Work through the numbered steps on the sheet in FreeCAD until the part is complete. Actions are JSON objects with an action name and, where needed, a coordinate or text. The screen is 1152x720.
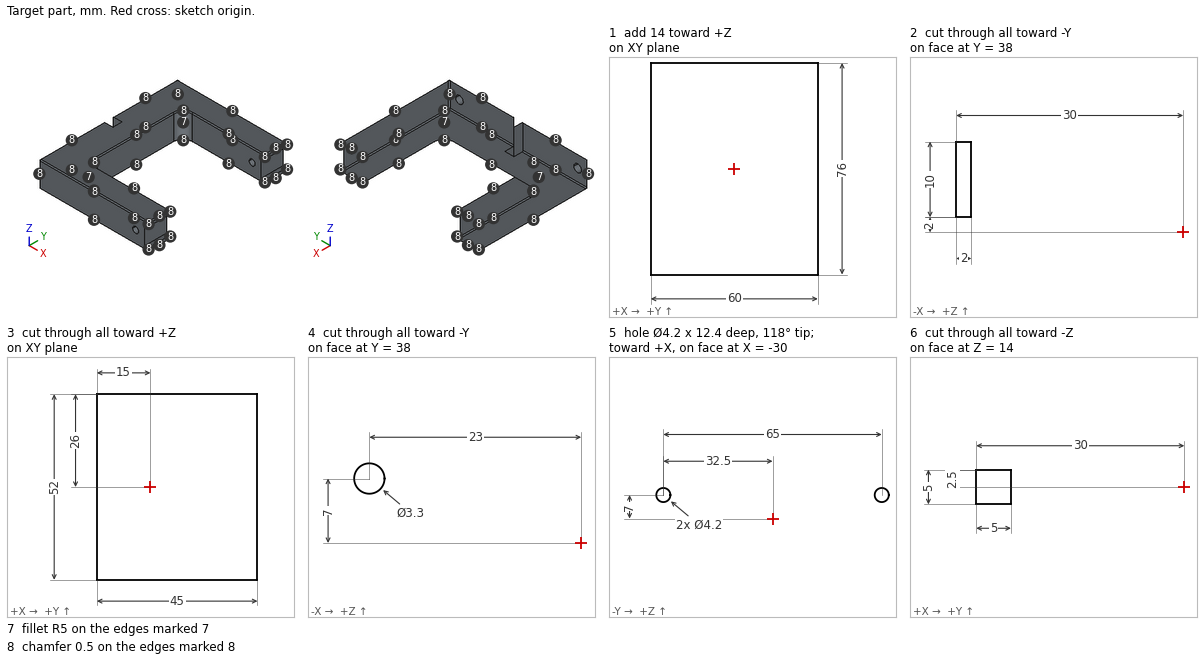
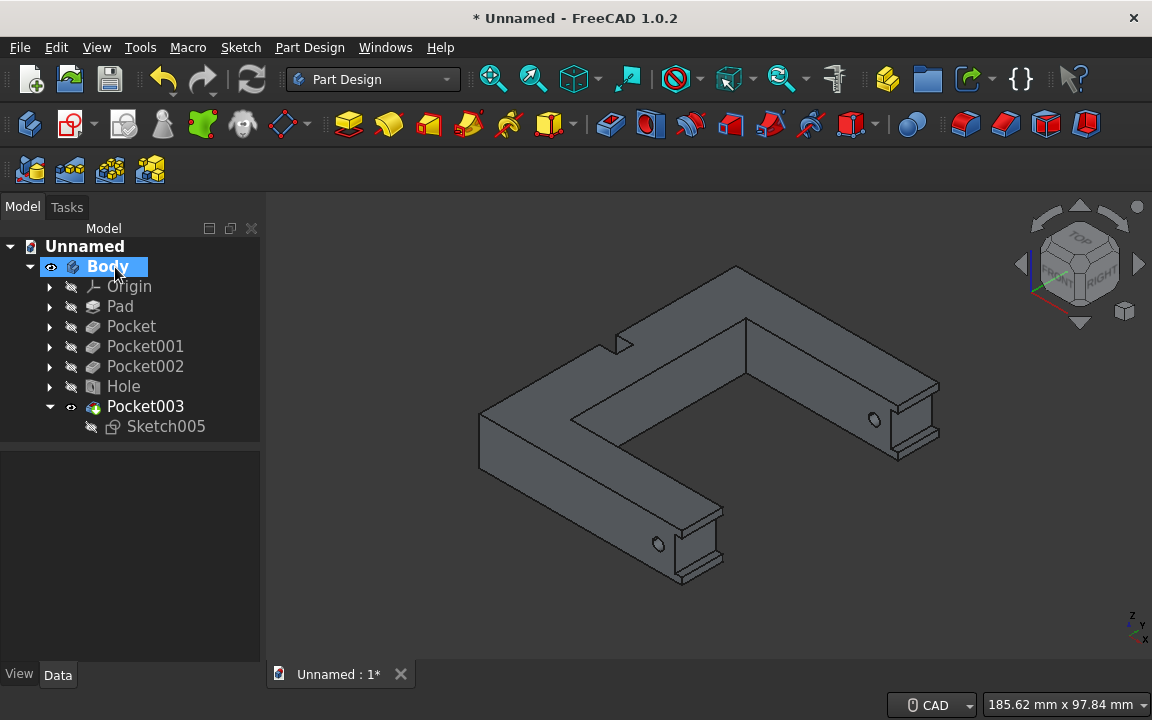
{"action": "key", "text": "1"}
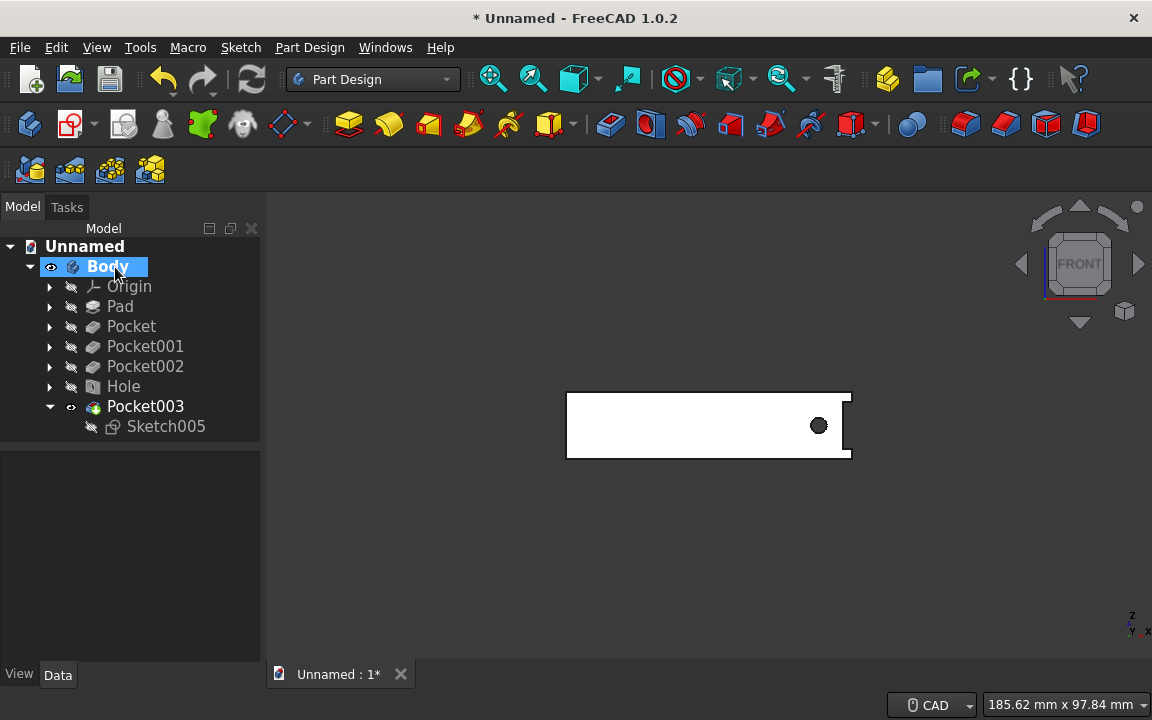
{"action": "key", "text": "v f"}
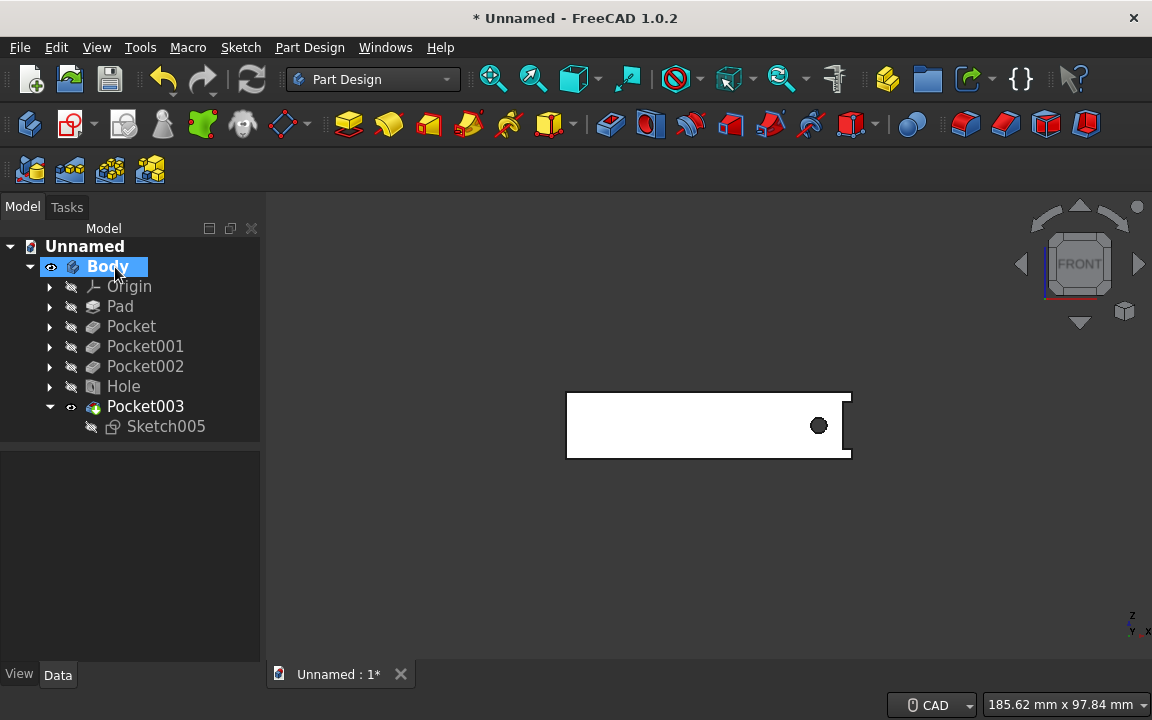
{"action": "key", "text": "3"}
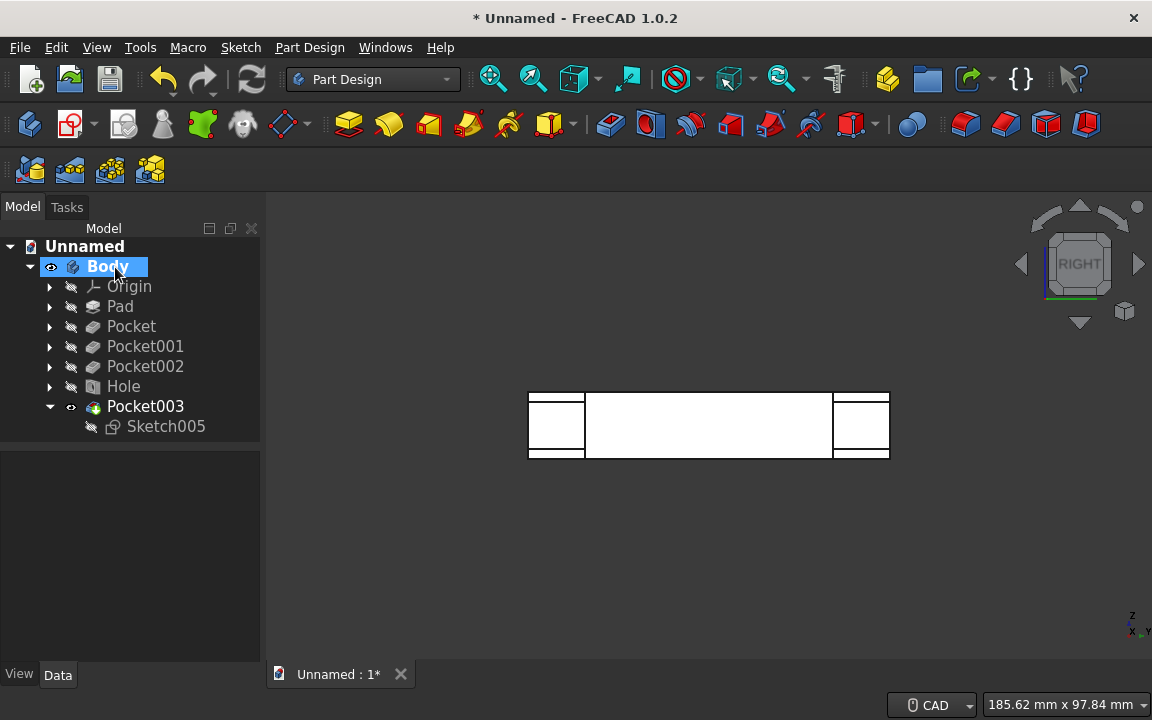
{"action": "key", "text": "v f"}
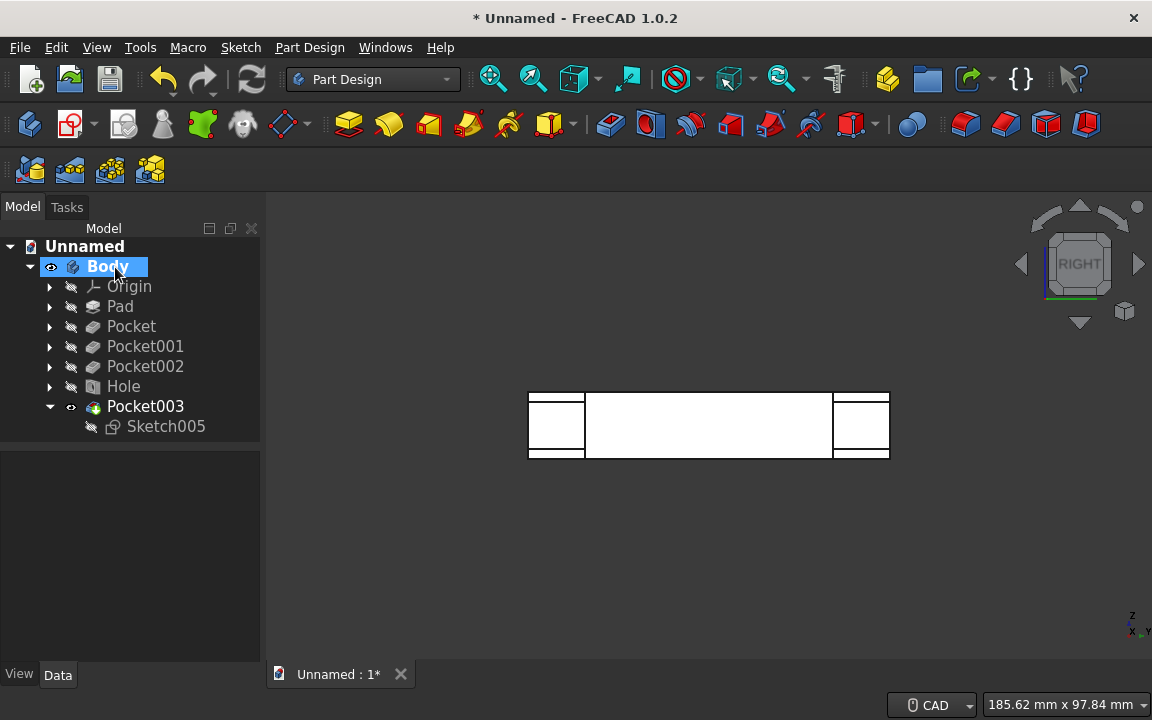
{"action": "key", "text": "5"}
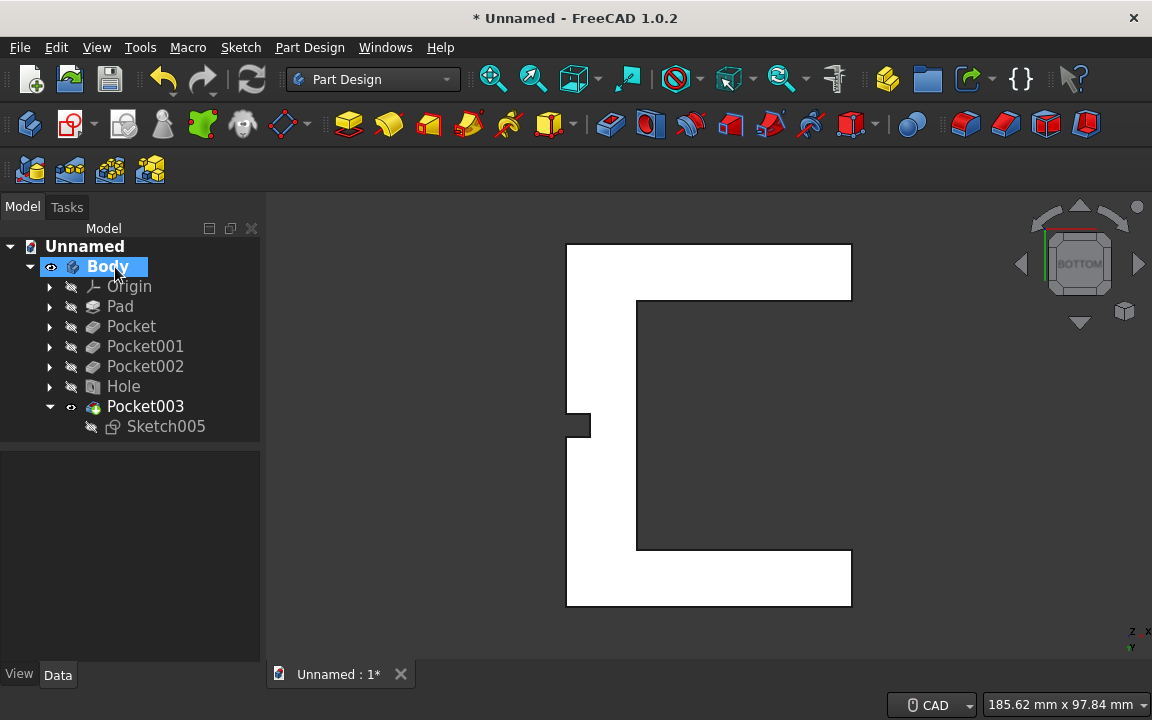
{"action": "key", "text": "4"}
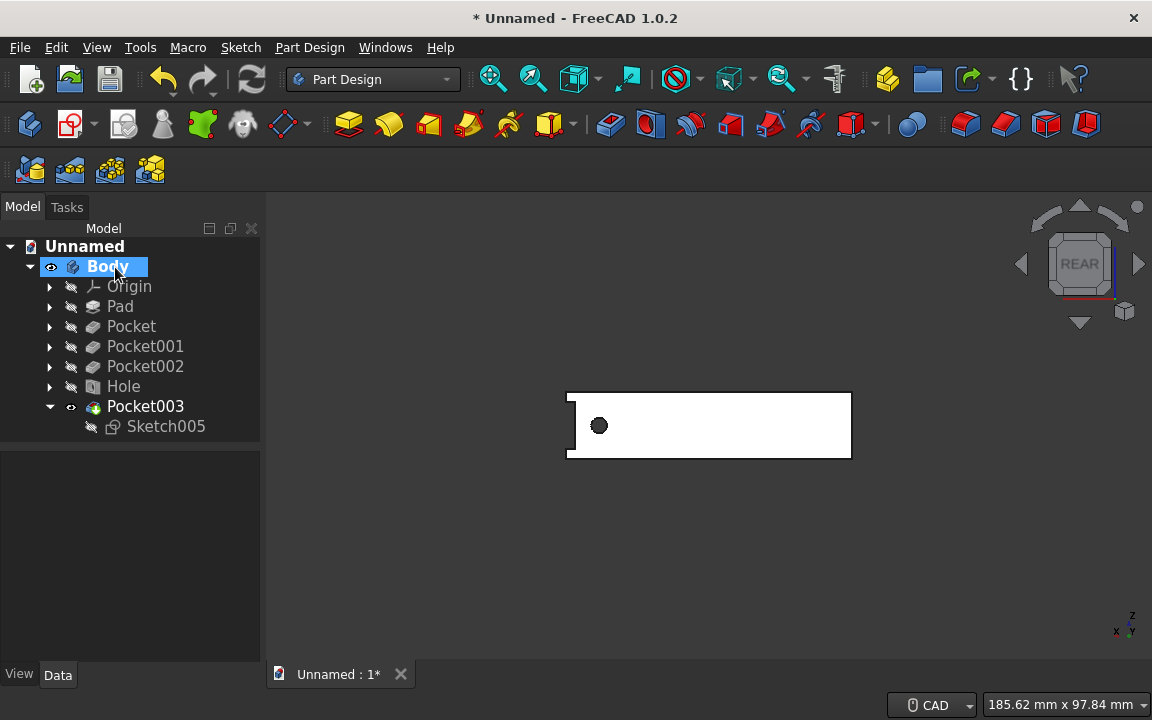
{"action": "key", "text": "v f"}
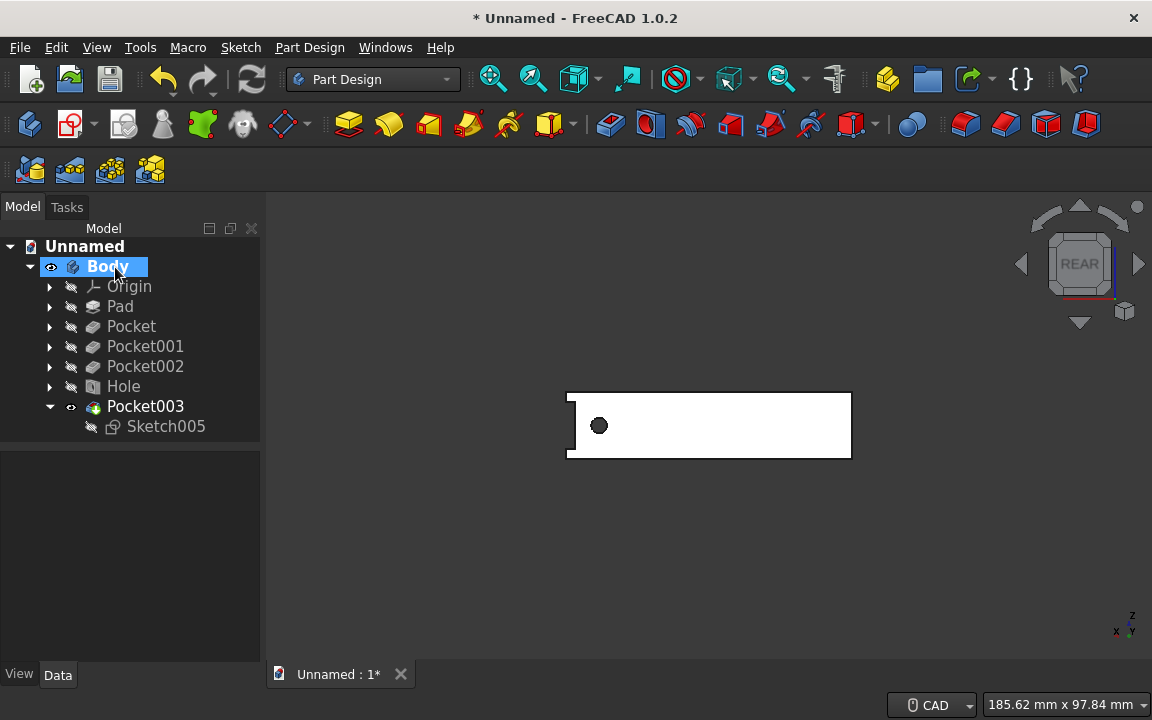
{"action": "key", "text": "6"}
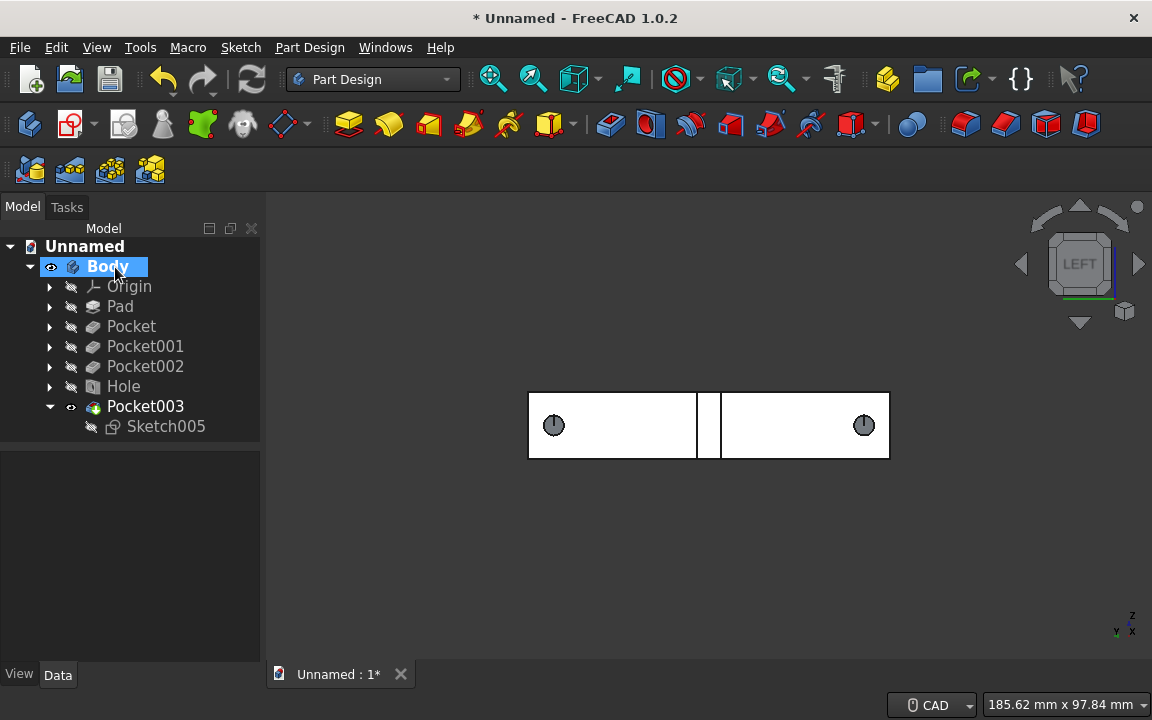
{"action": "key", "text": "v f"}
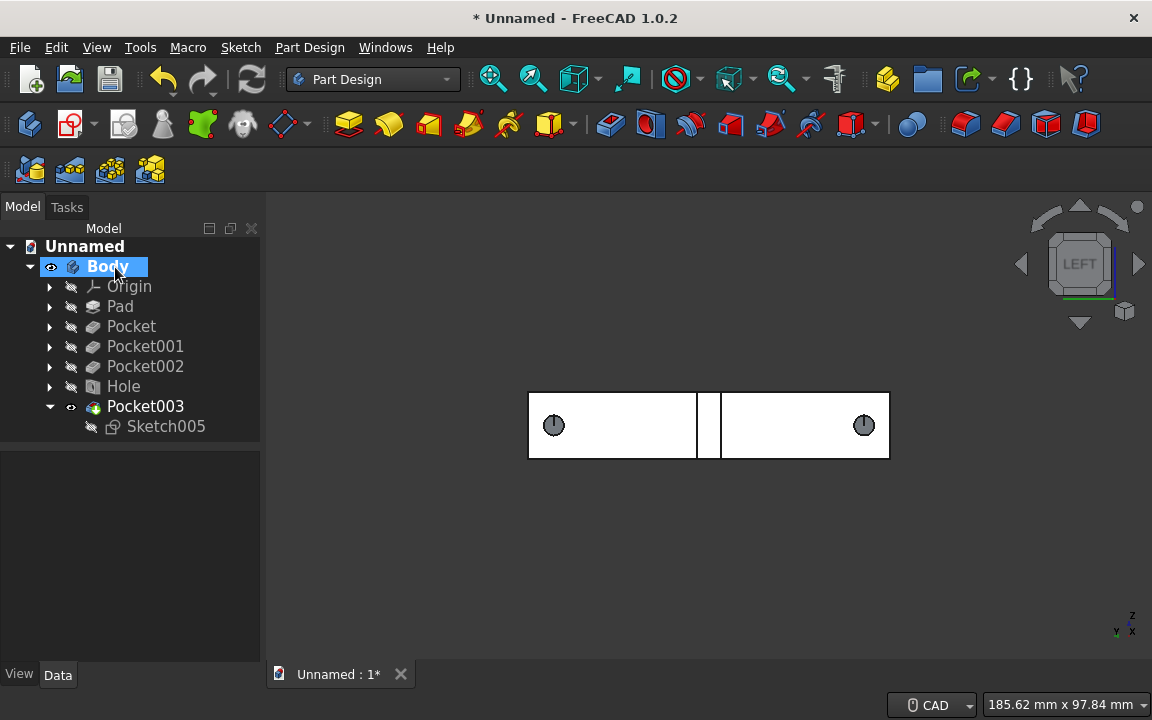
{"action": "key", "text": "v 3"}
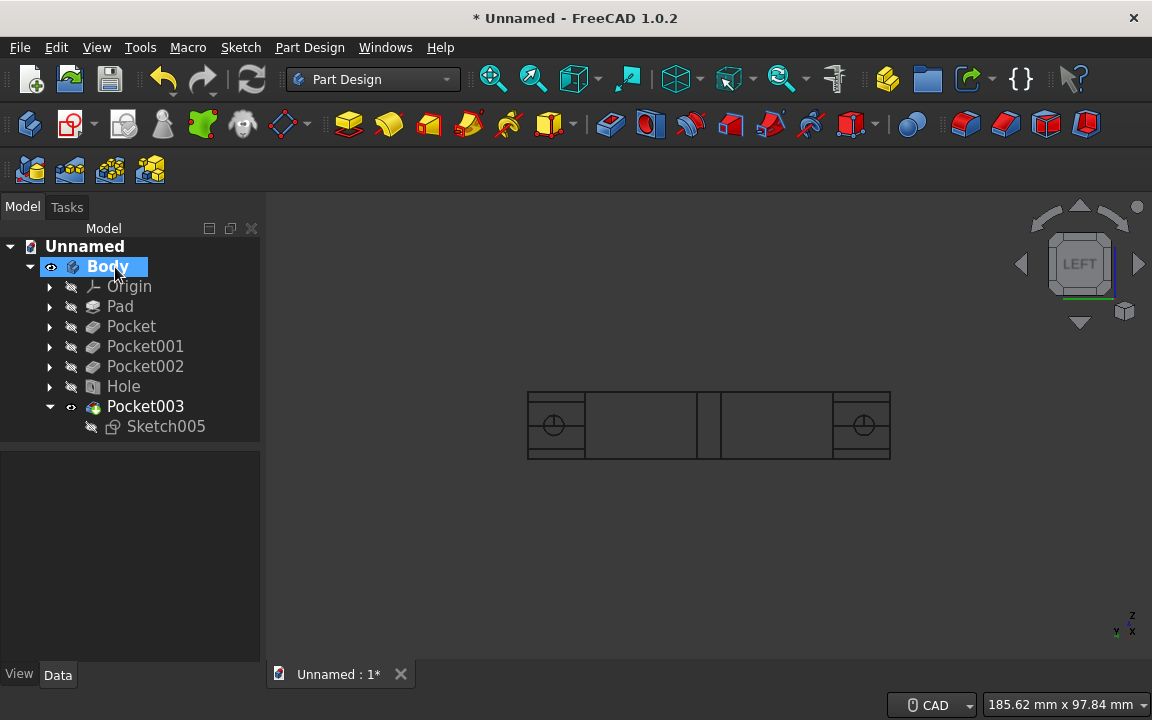
{"action": "key", "text": "0"}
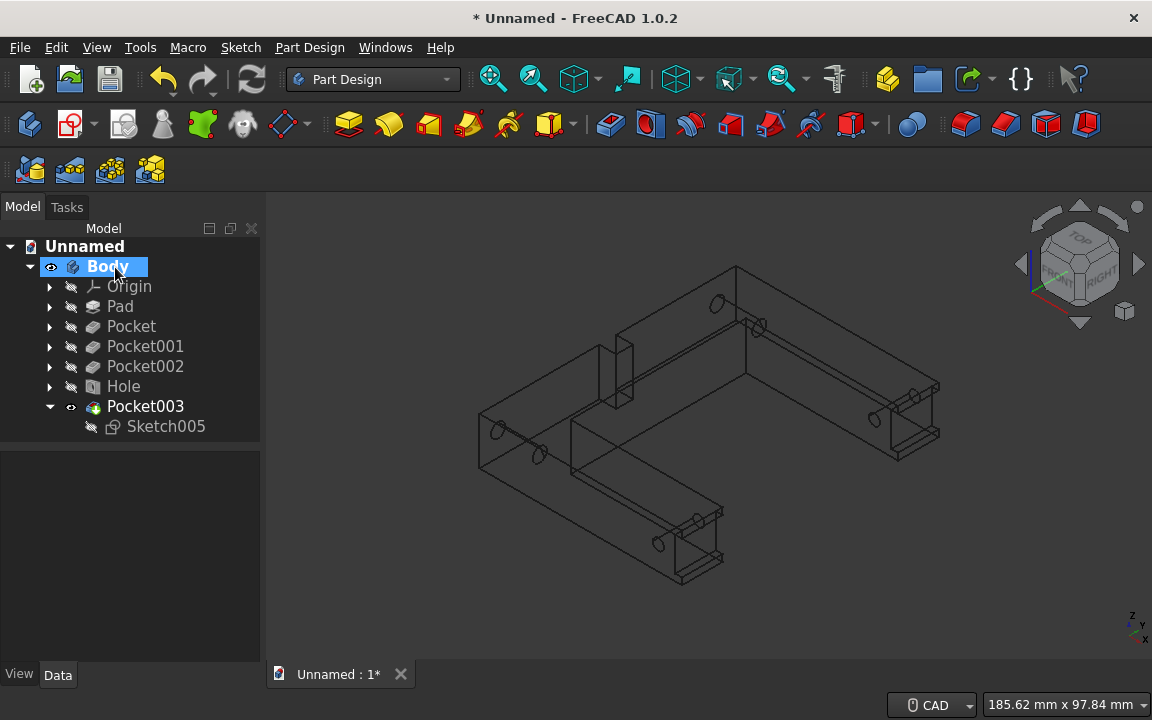
{"action": "left_click", "coordinate": [571, 446]}